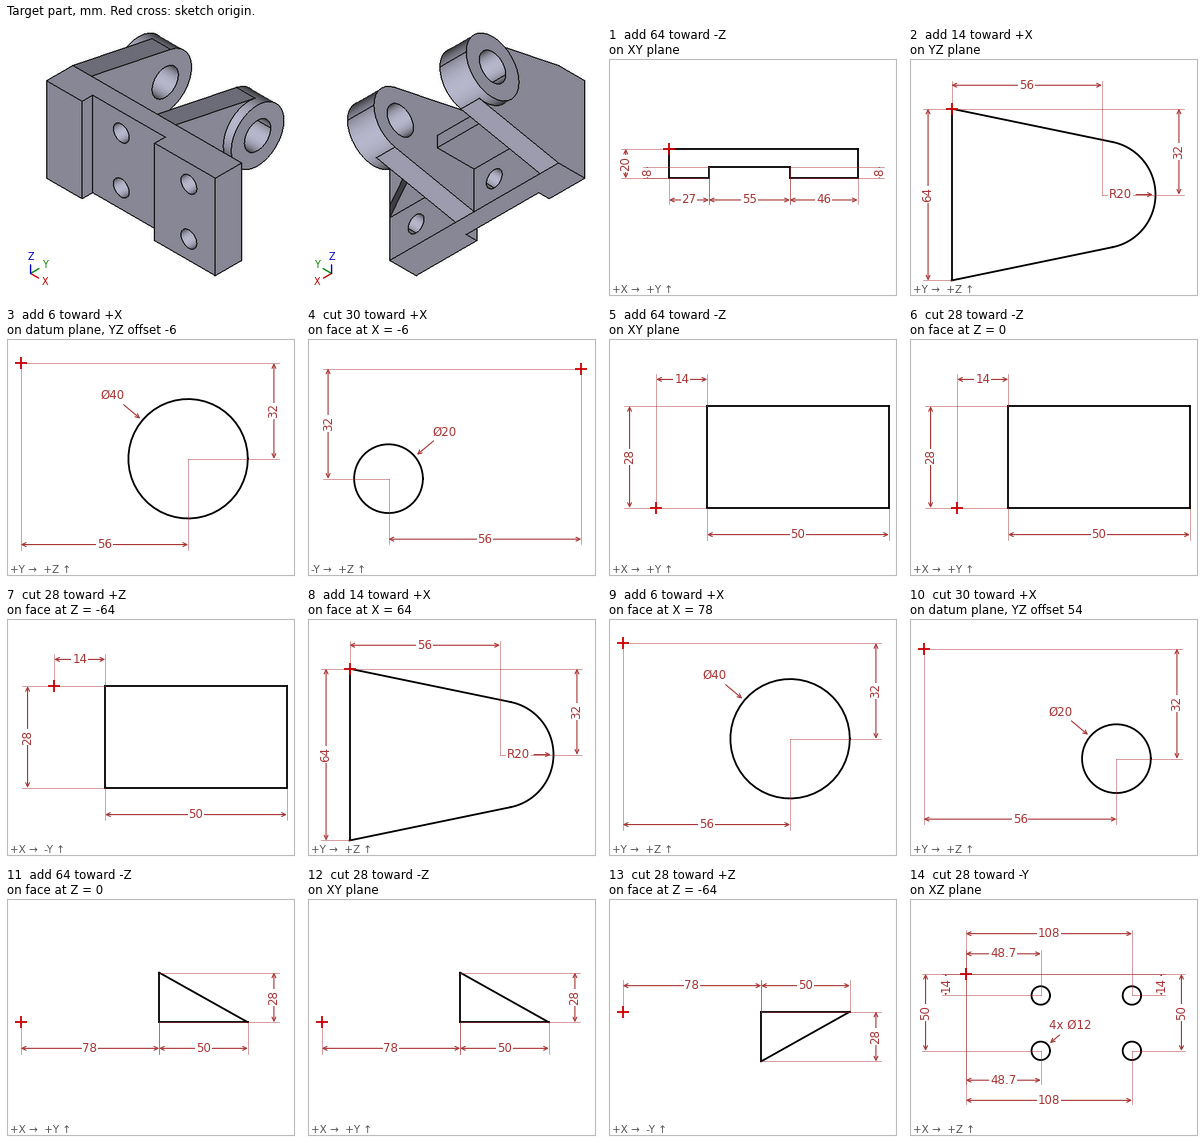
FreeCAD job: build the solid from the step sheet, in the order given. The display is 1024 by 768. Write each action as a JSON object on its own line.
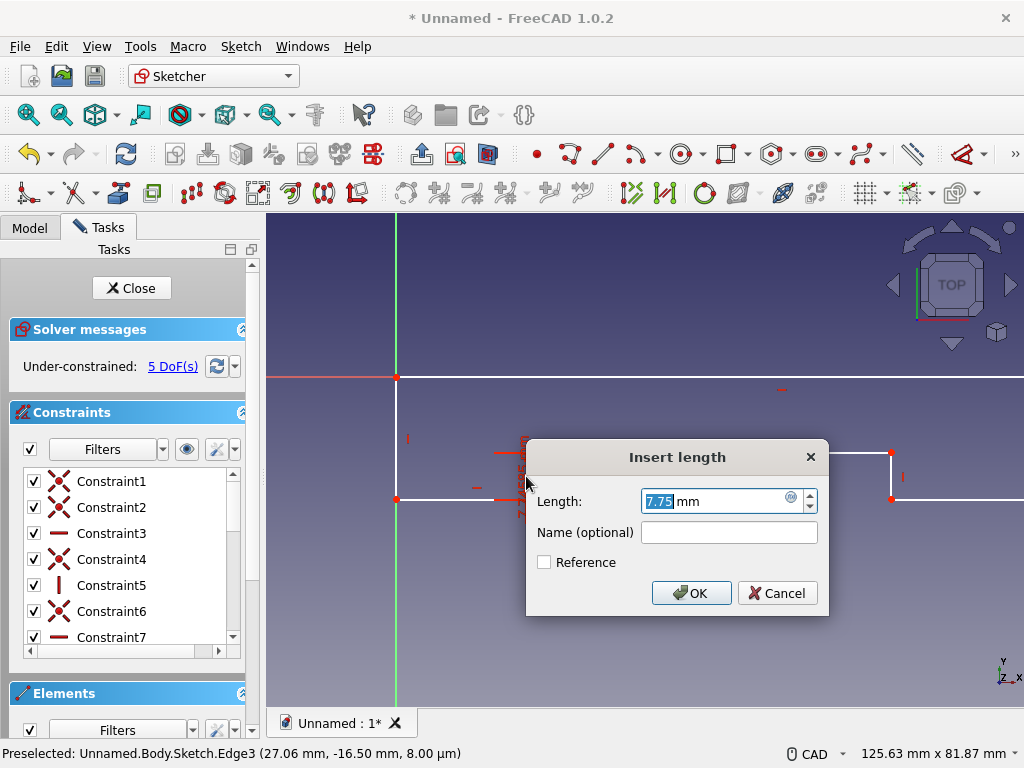
{"action": "type", "text": "8"}
{"action": "key", "text": "Return"}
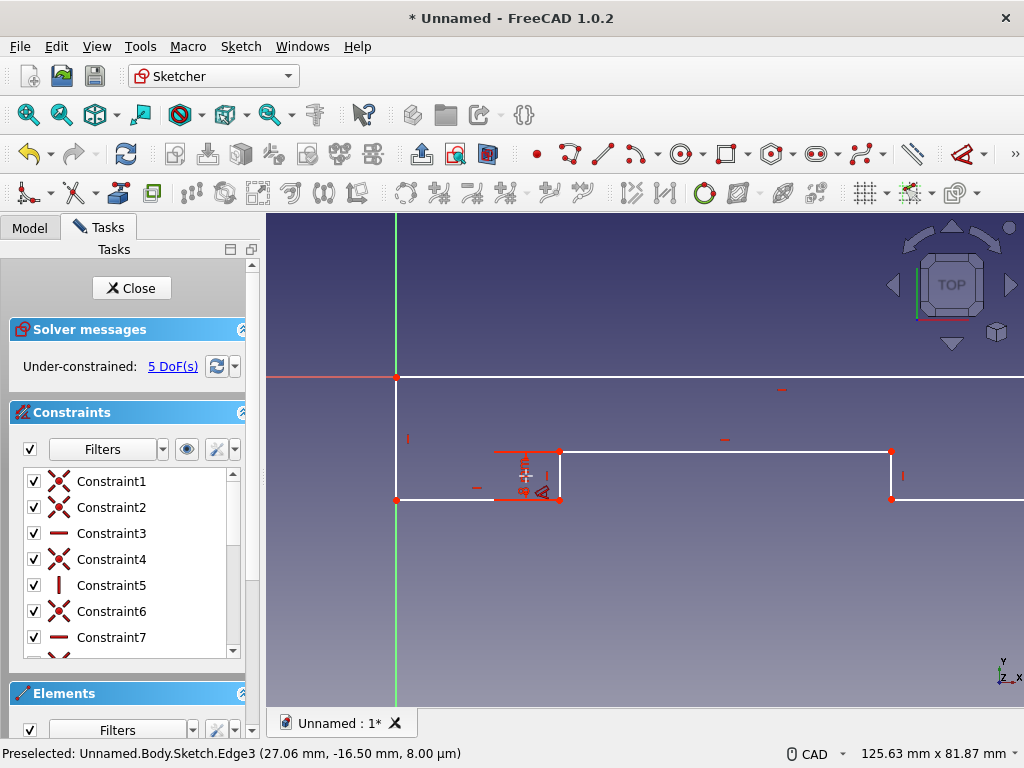
{"action": "scroll", "coordinate": [326, 487], "scroll_direction": "down", "scroll_amount": 3}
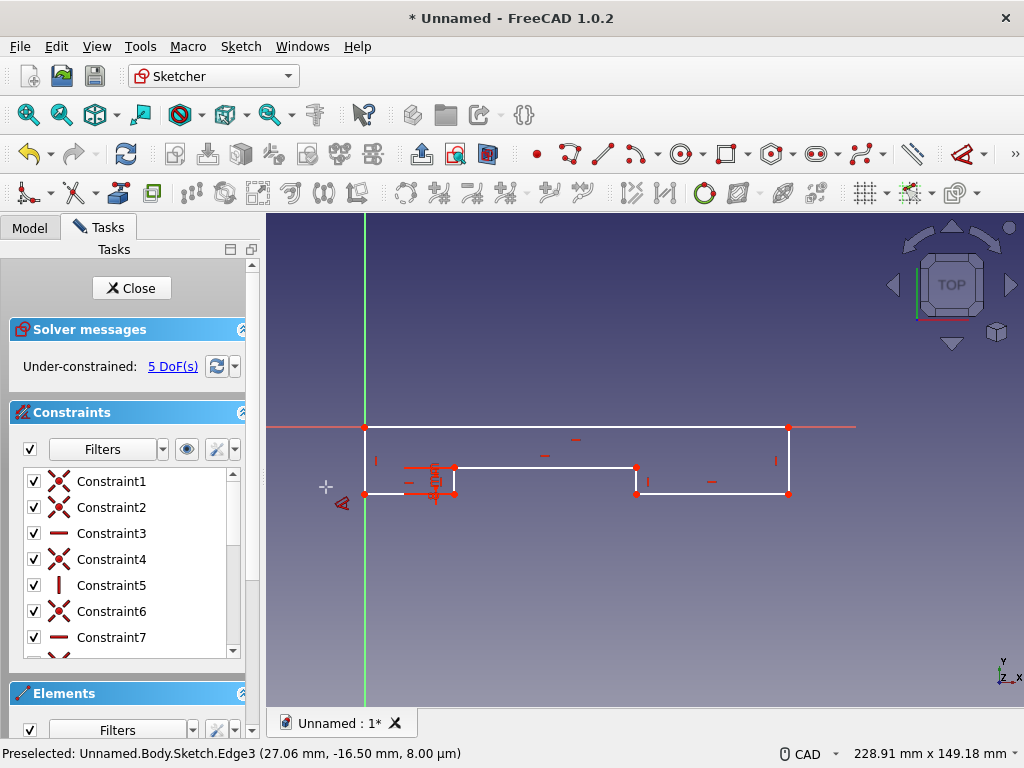
{"action": "scroll", "coordinate": [636, 476], "scroll_direction": "up", "scroll_amount": 3}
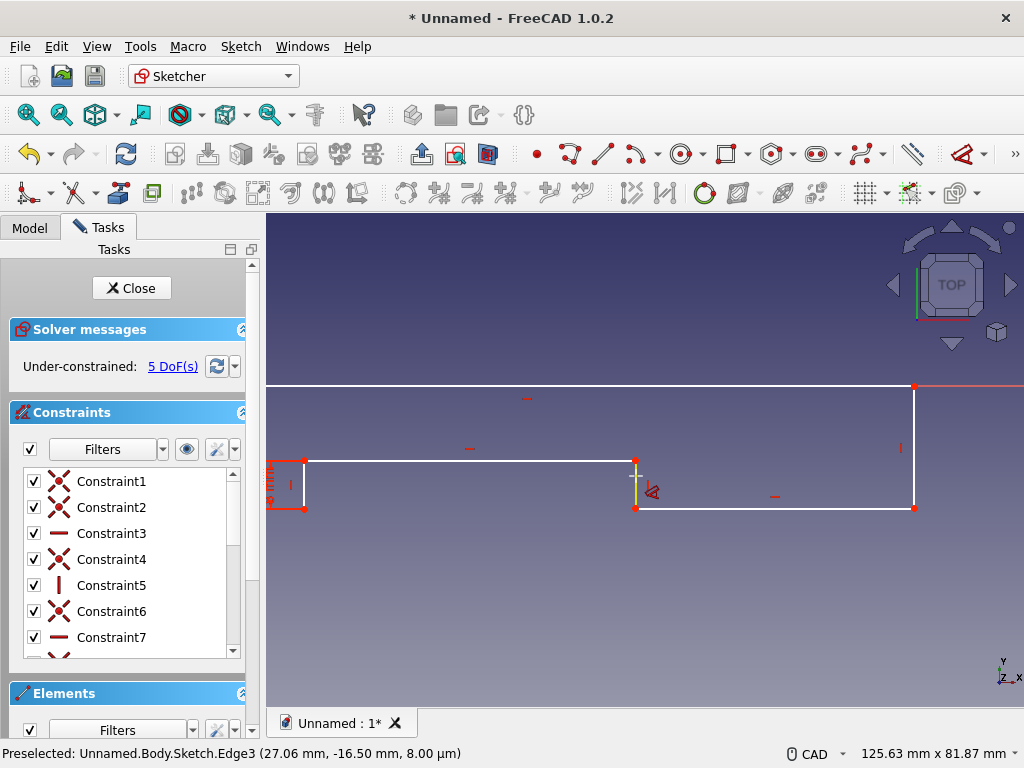
{"action": "left_click", "coordinate": [636, 475]}
{"action": "left_click", "coordinate": [670, 485]}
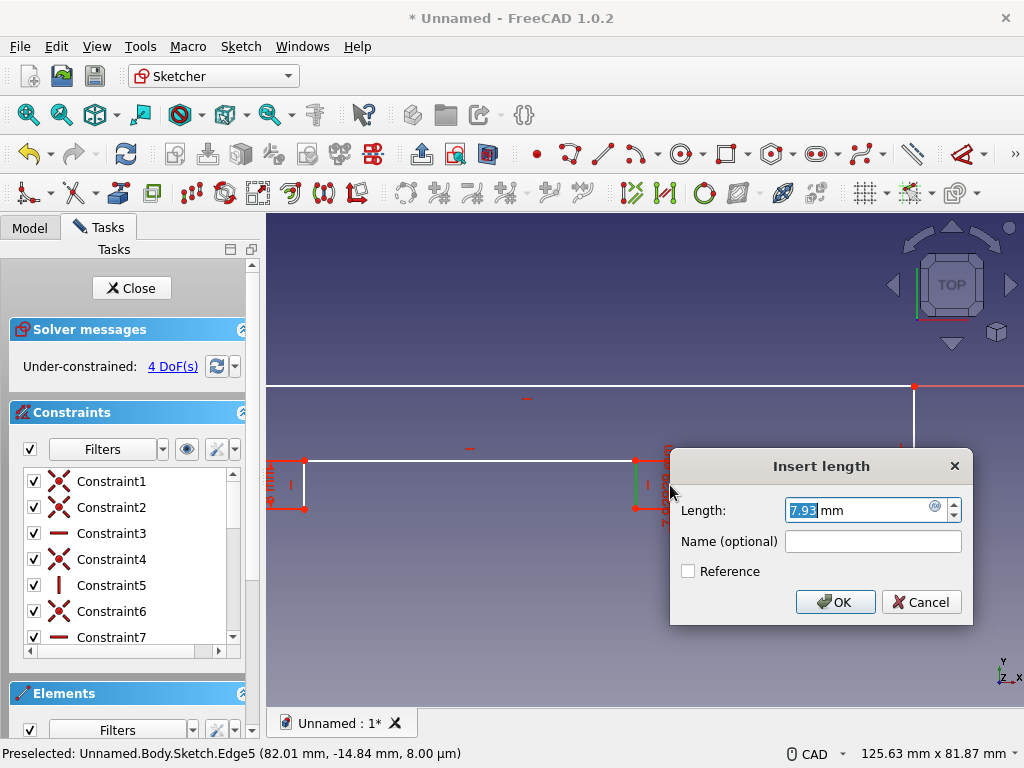
{"action": "type", "text": "8"}
{"action": "key", "text": "Return"}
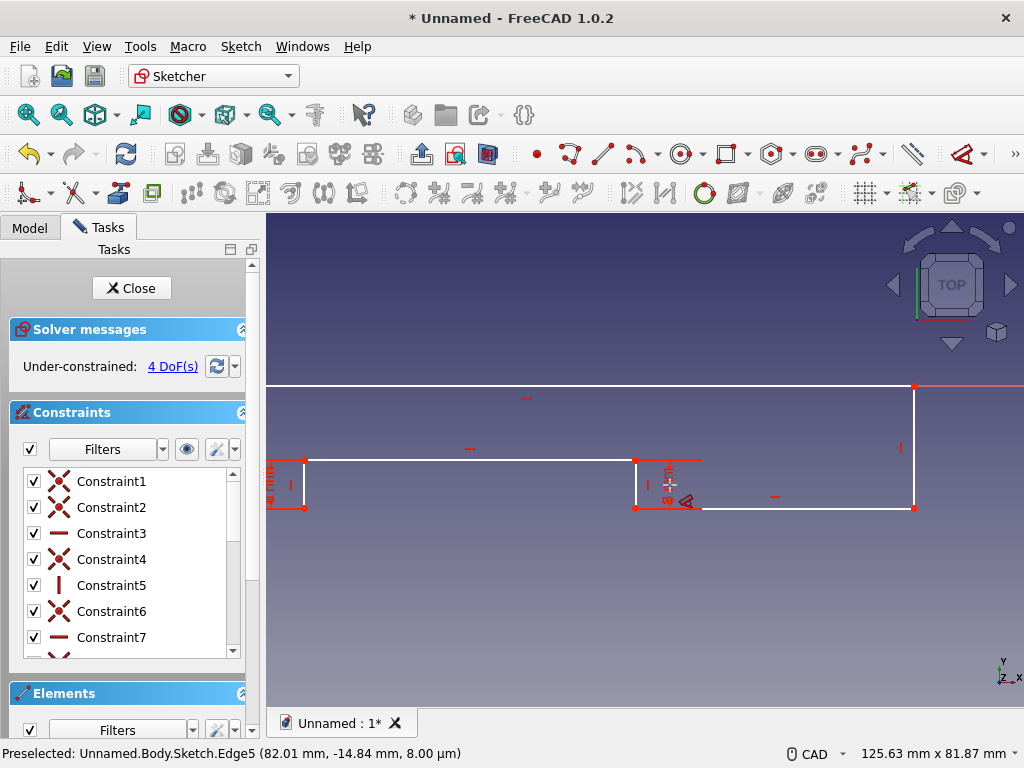
{"action": "scroll", "coordinate": [636, 476], "scroll_direction": "down", "scroll_amount": 3}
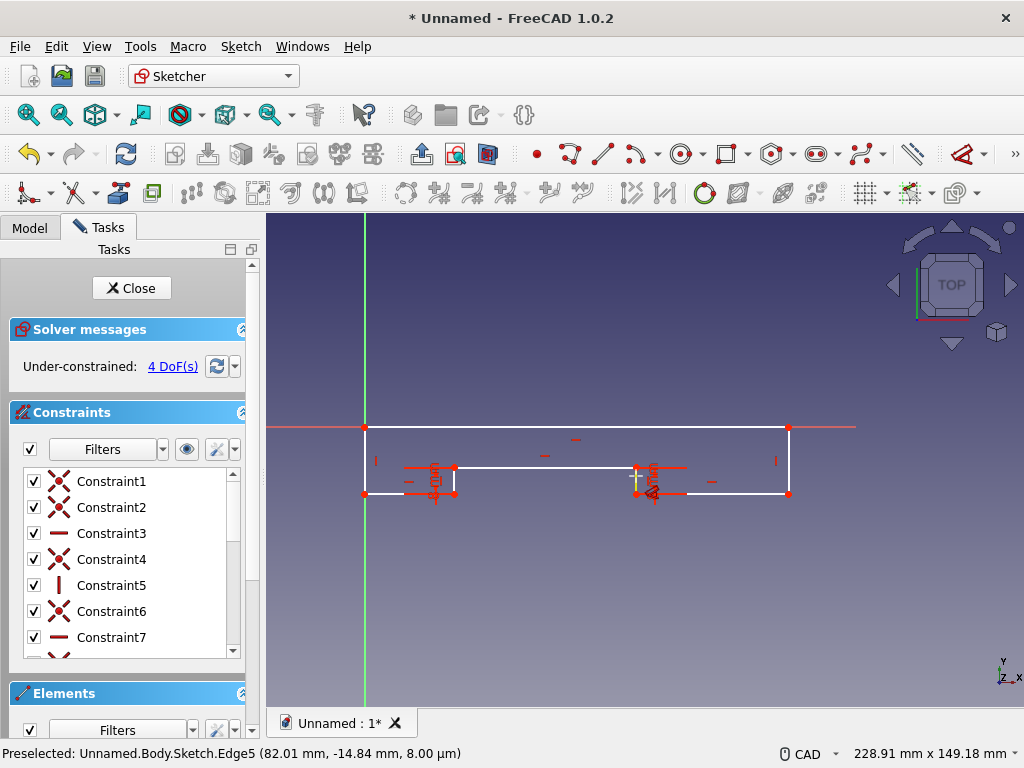
{"action": "left_click", "coordinate": [365, 447]}
{"action": "left_click", "coordinate": [331, 461]}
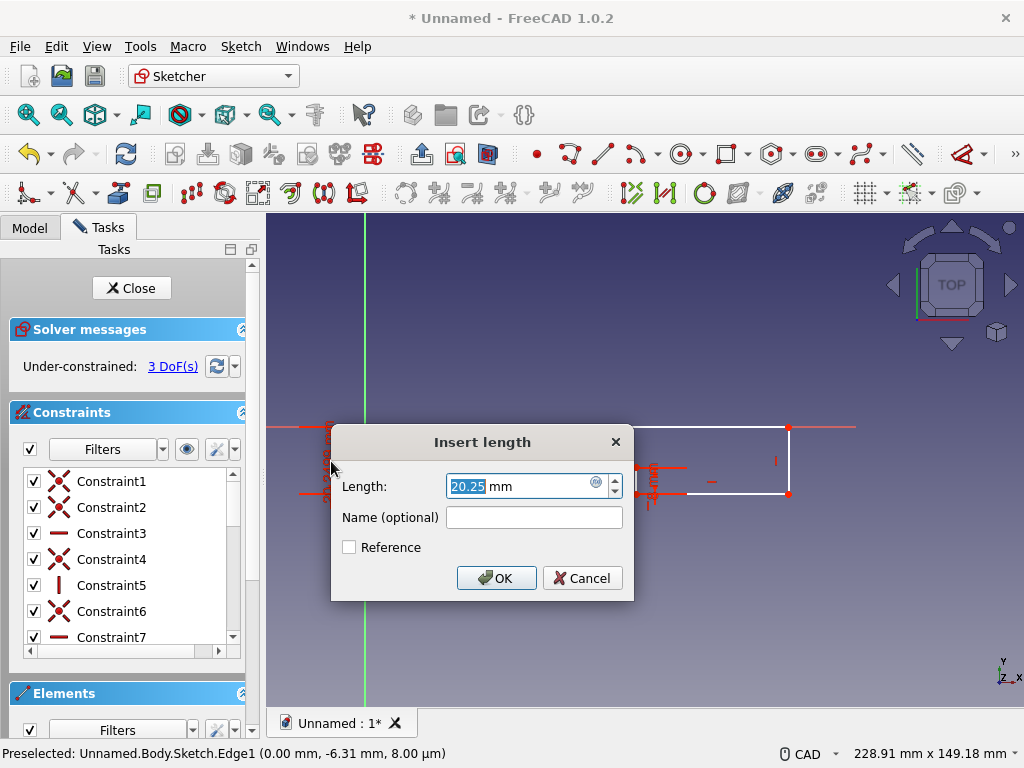
{"action": "type", "text": "20"}
{"action": "key", "text": "Return"}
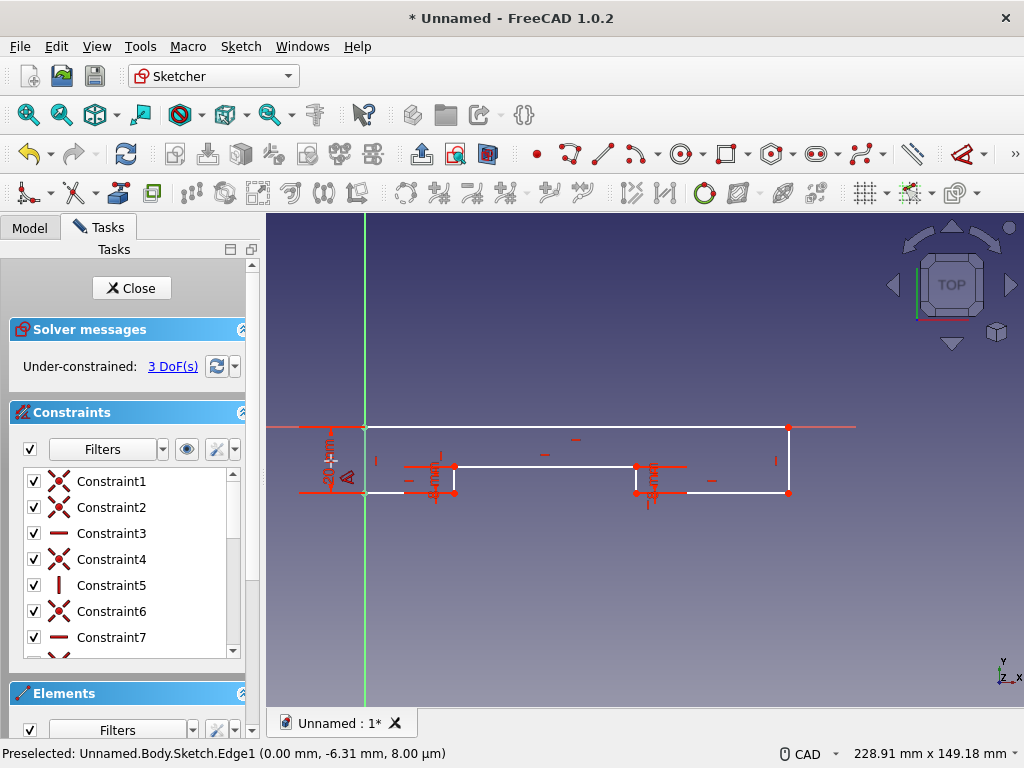
{"action": "left_click", "coordinate": [391, 493]}
{"action": "left_click", "coordinate": [409, 527]}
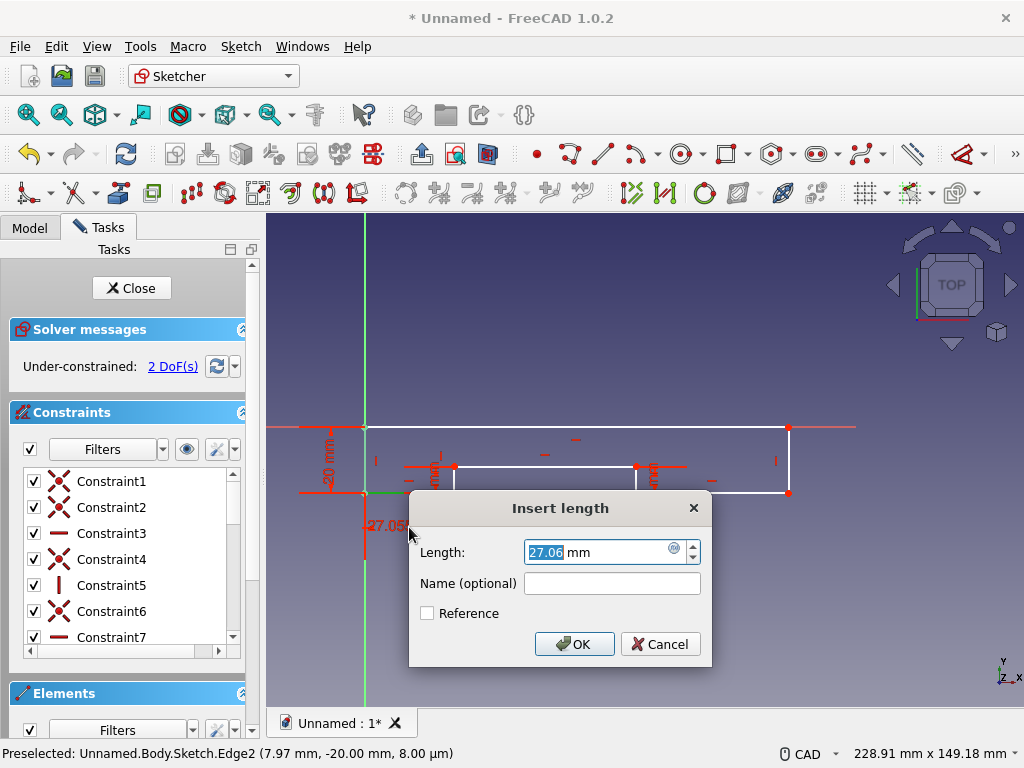
{"action": "type", "text": "27"}
{"action": "key", "text": "Return"}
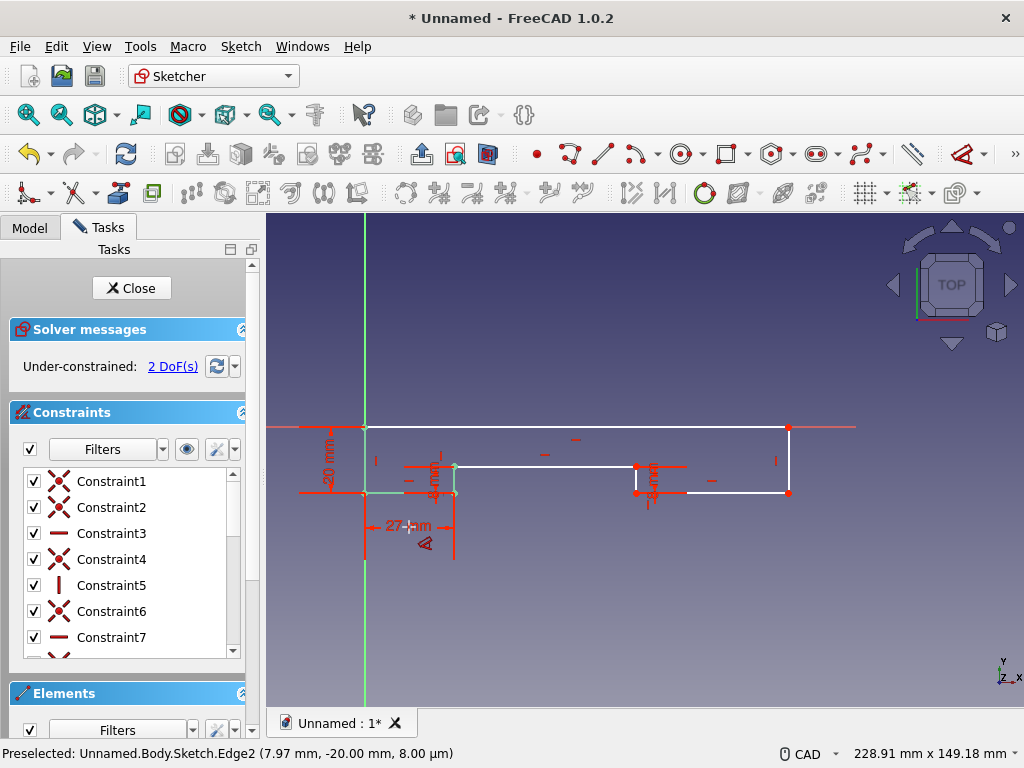
{"action": "left_click", "coordinate": [509, 467]}
{"action": "left_click", "coordinate": [545, 501]}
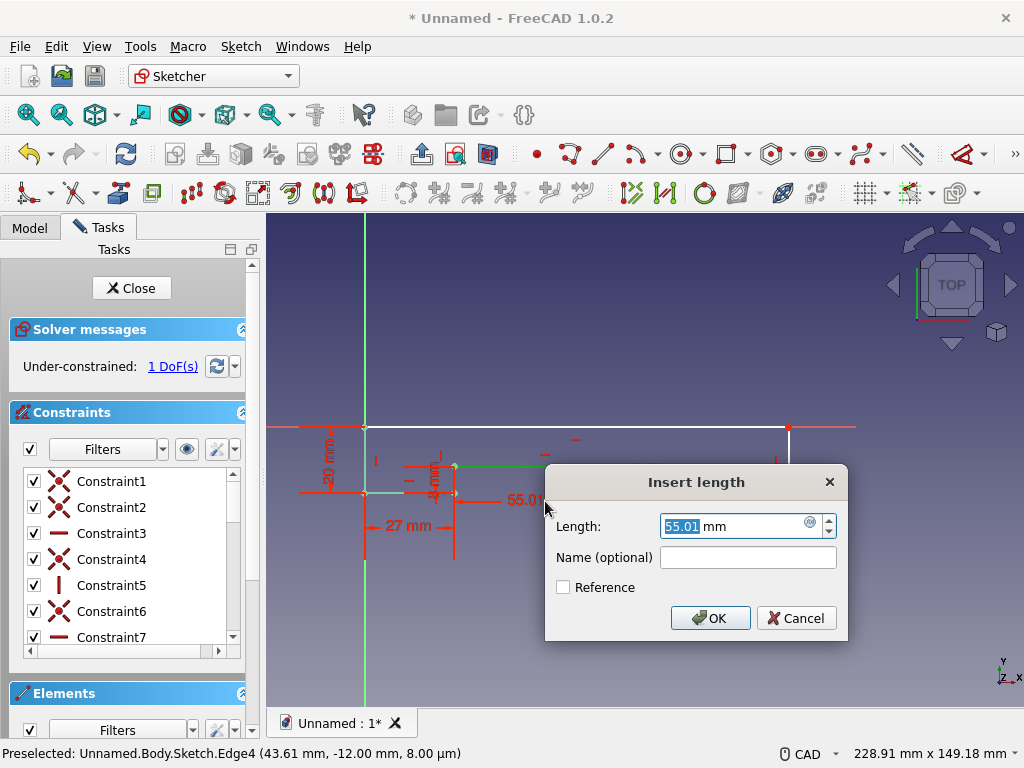
{"action": "type", "text": "55"}
{"action": "key", "text": "Return"}